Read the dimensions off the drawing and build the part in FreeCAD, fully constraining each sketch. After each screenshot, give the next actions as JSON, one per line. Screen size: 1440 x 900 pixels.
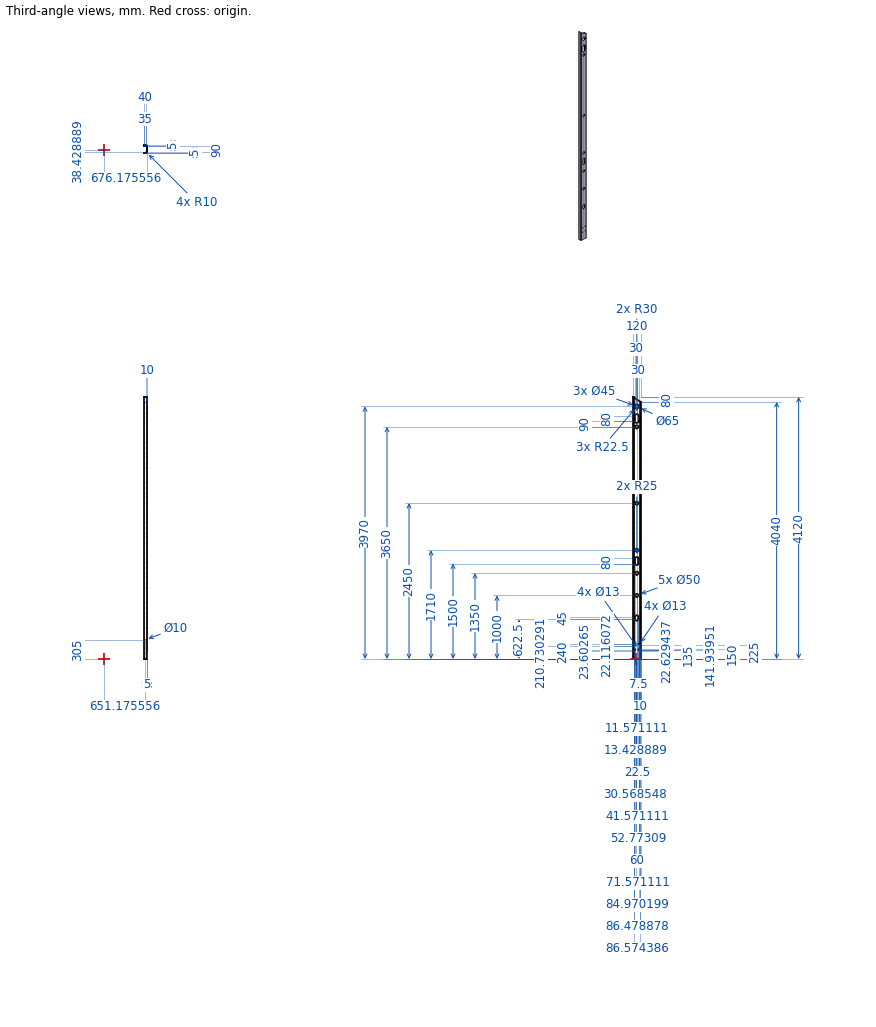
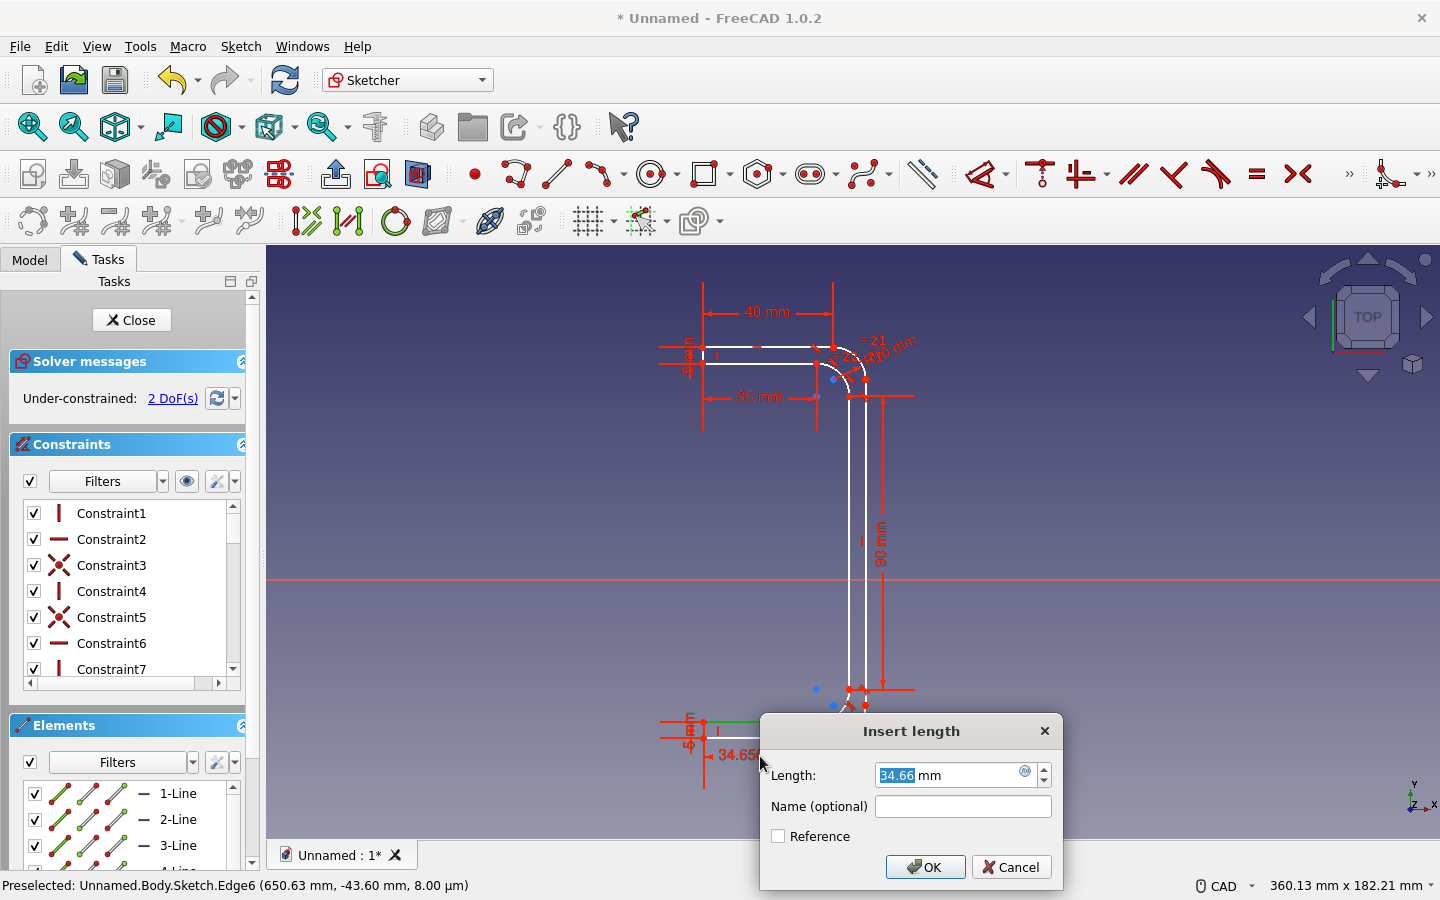
{"action": "type", "text": "35"}
{"action": "key", "text": "Return"}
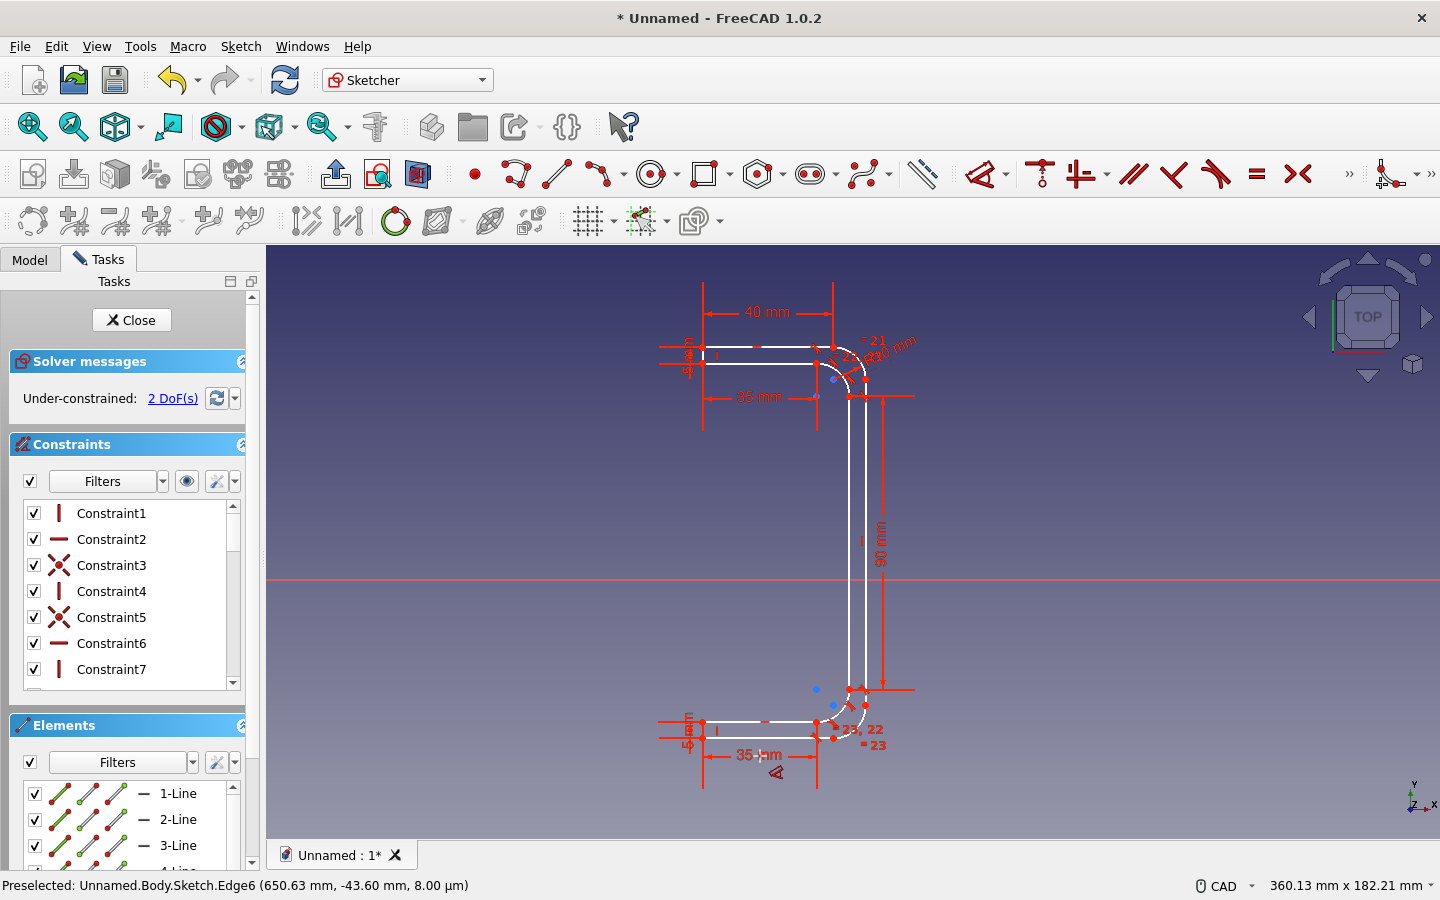
{"action": "left_click", "coordinate": [866, 706]}
{"action": "left_click", "coordinate": [900, 643]}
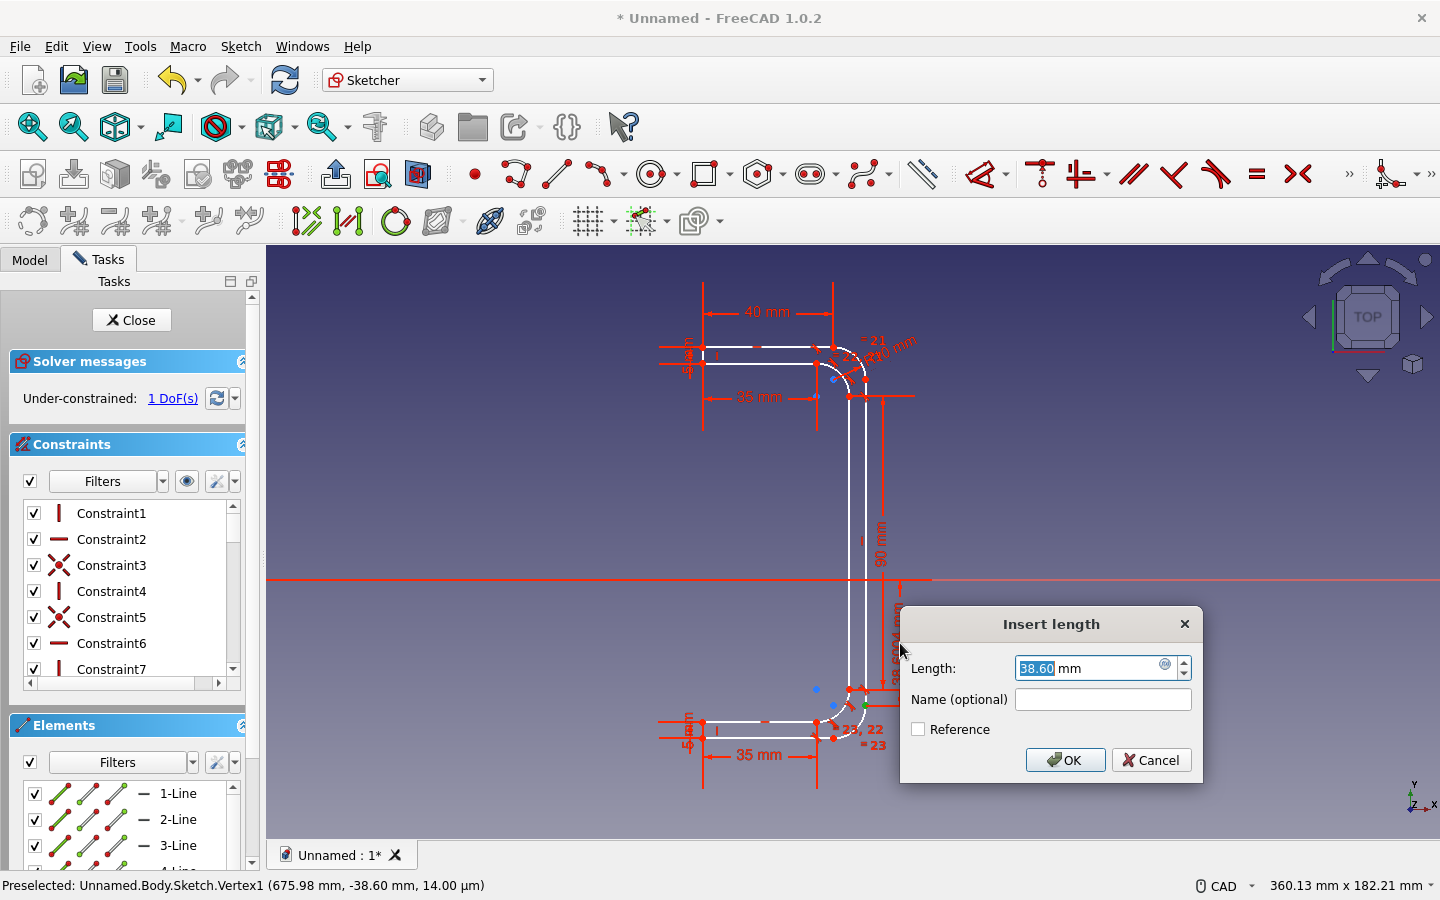
{"action": "type", "text": "38.428889"}
{"action": "key", "text": "Return"}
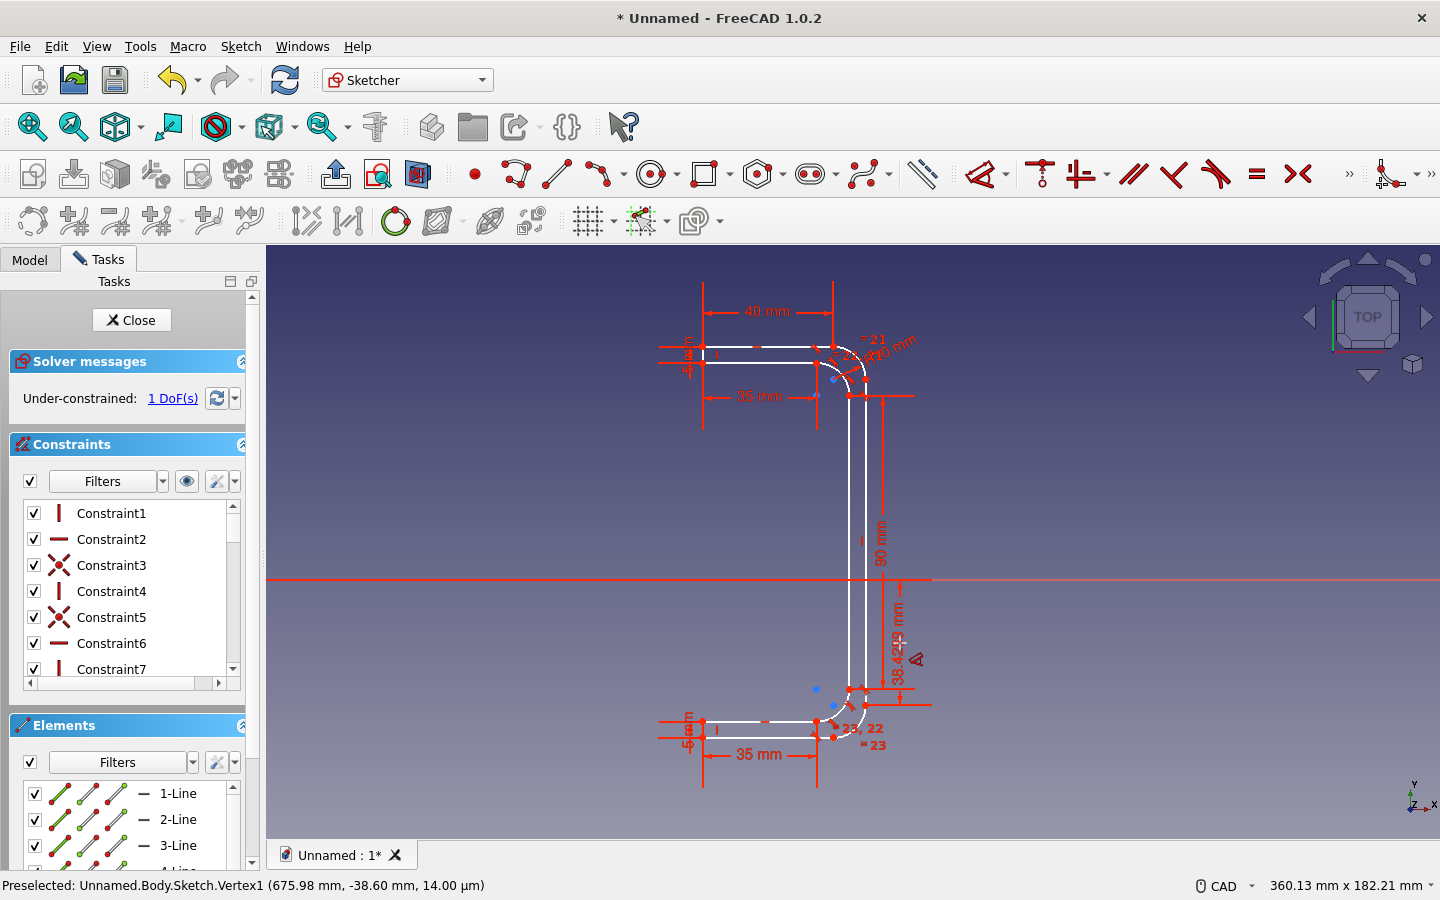
{"action": "left_click", "coordinate": [866, 705]}
{"action": "left_click", "coordinate": [580, 739]}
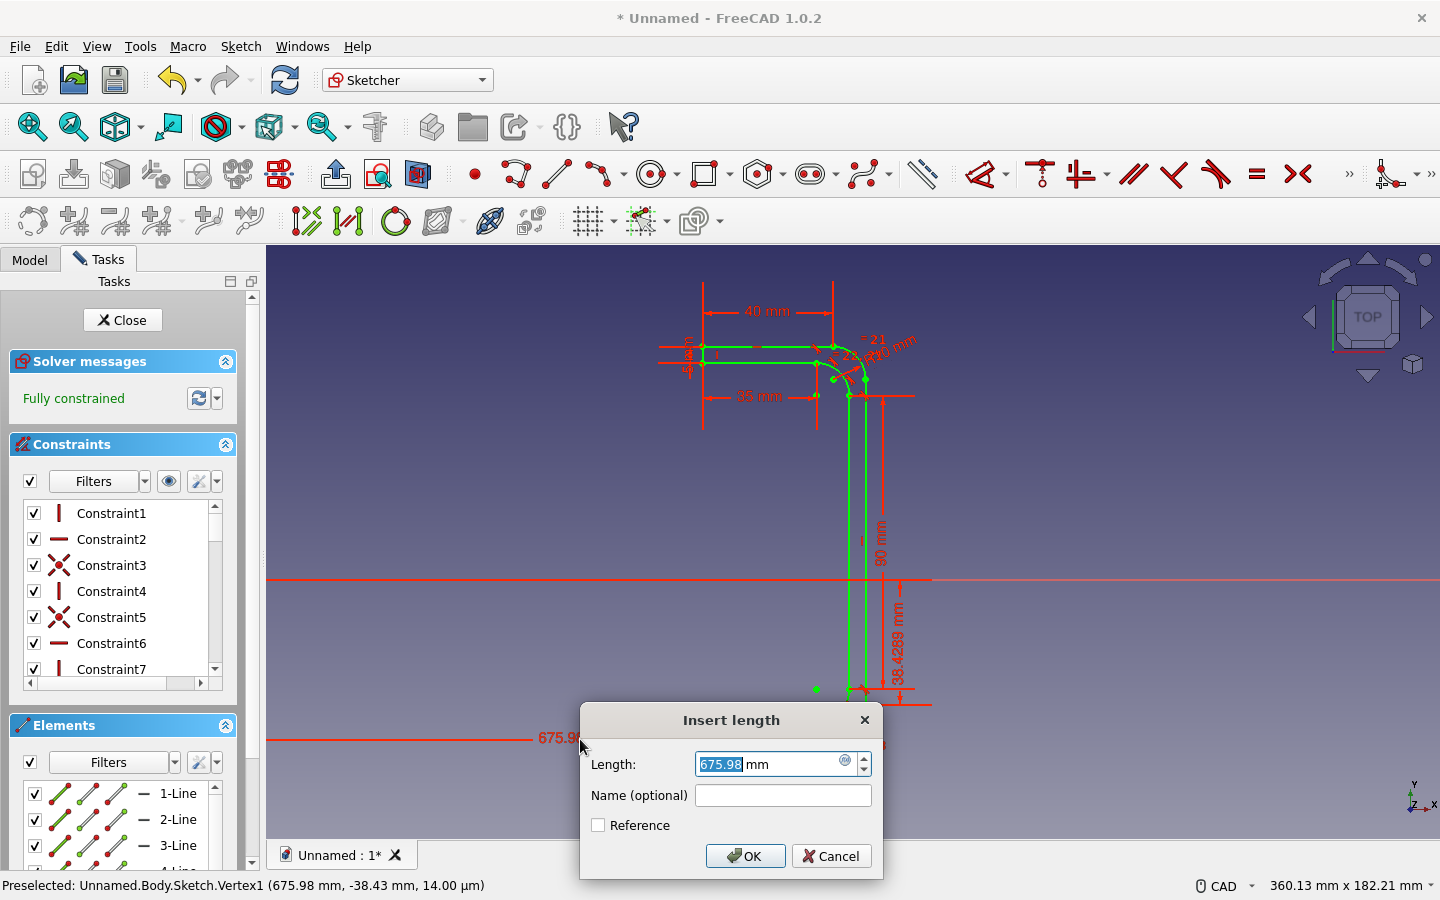
{"action": "type", "text": "676.175556"}
{"action": "key", "text": "Return"}
{"action": "key", "text": "Escape"}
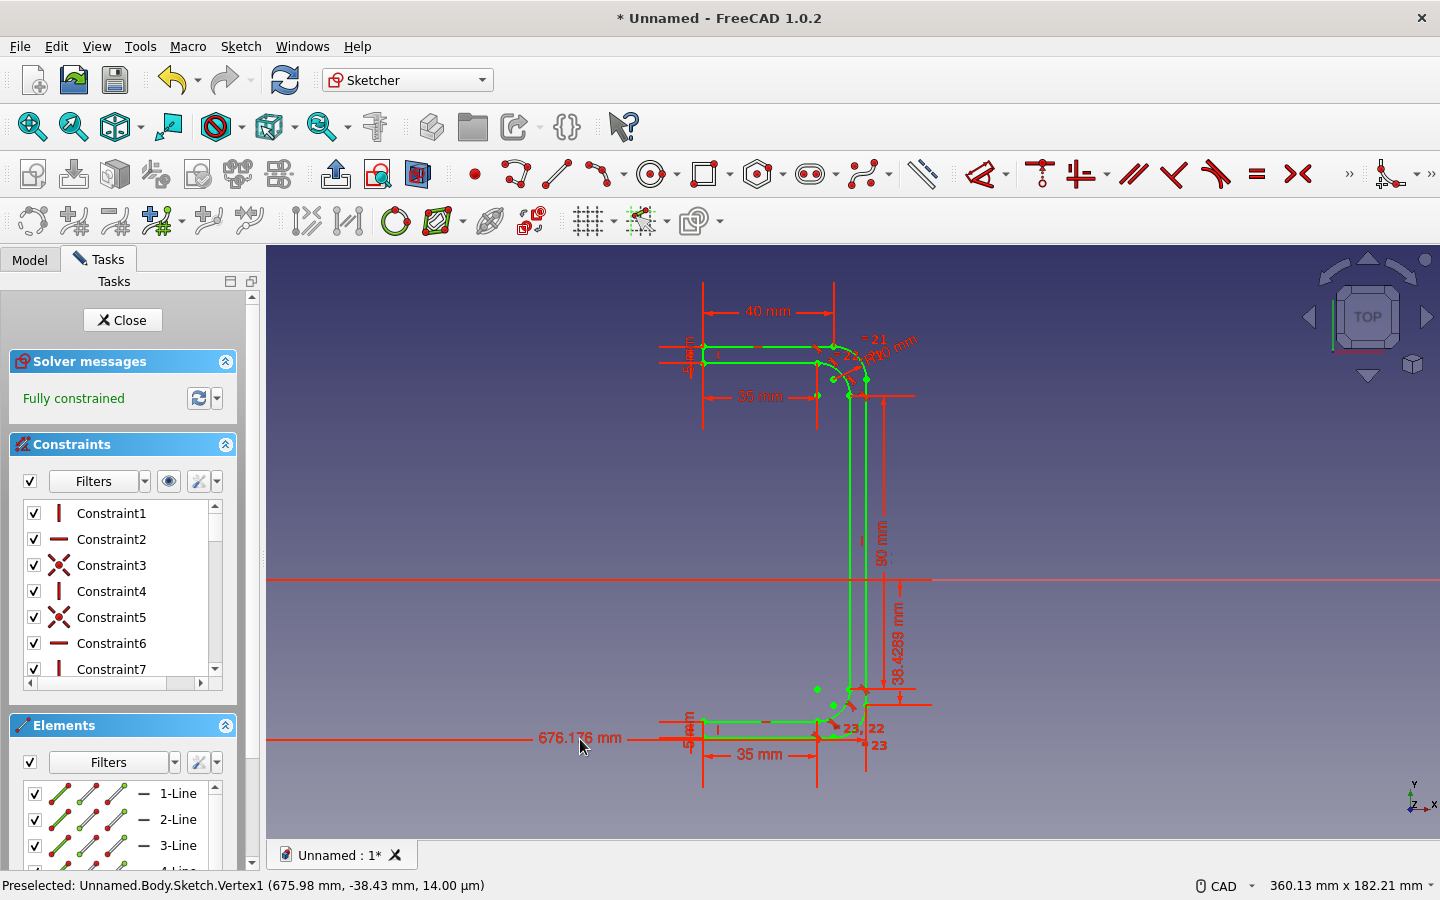
{"action": "left_click", "coordinate": [123, 320]}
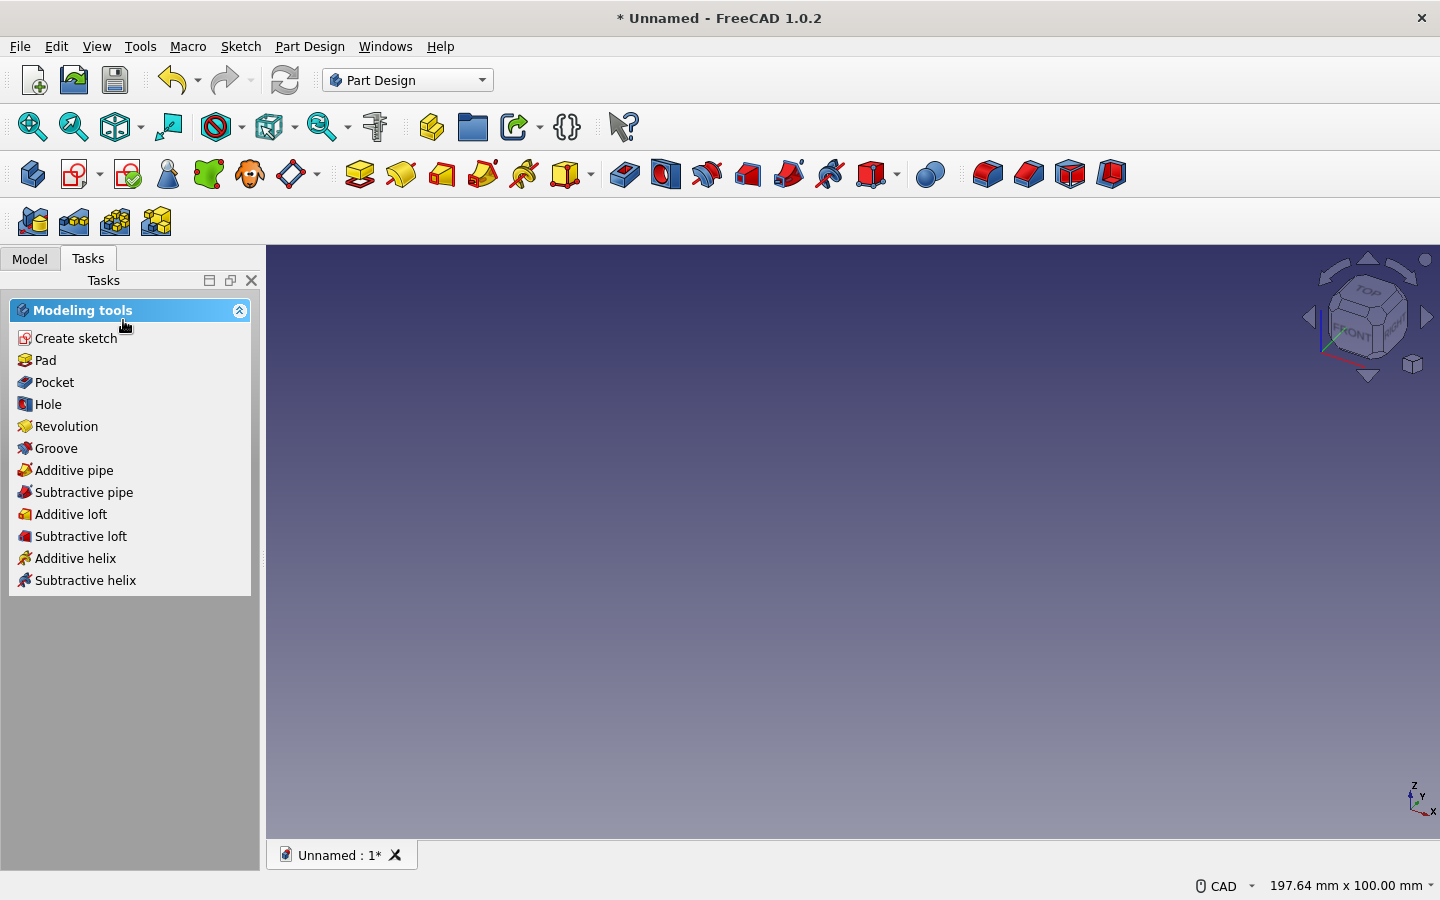
{"action": "left_click", "coordinate": [360, 174]}